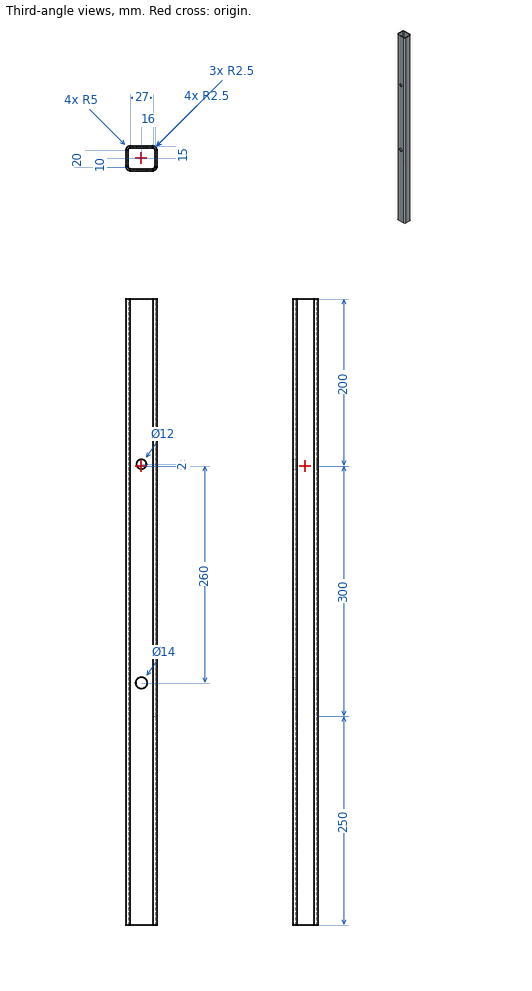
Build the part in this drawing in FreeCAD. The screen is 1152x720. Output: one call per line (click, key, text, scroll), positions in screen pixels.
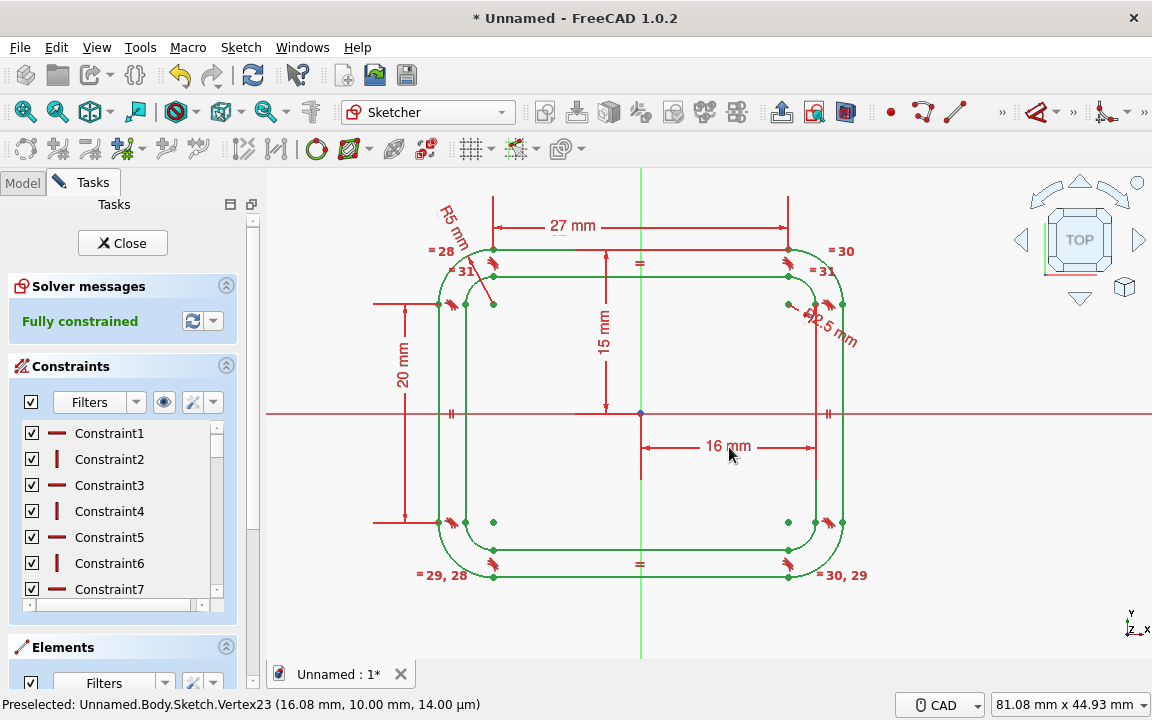
click(123, 243)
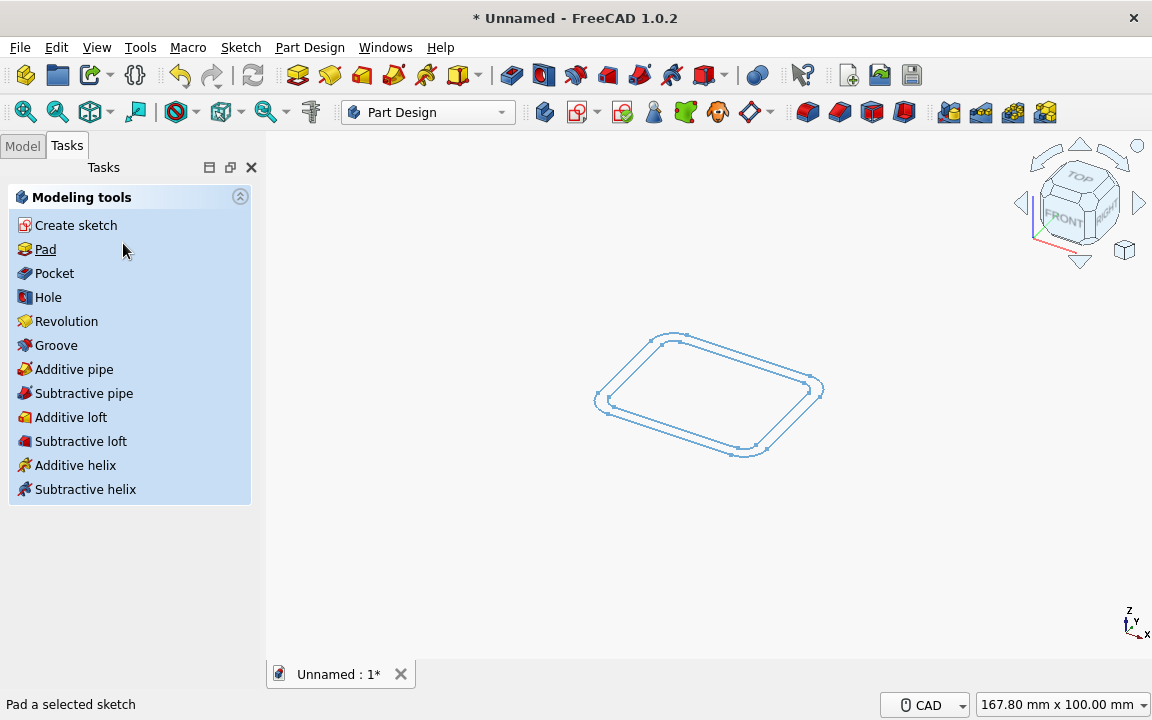
click(298, 76)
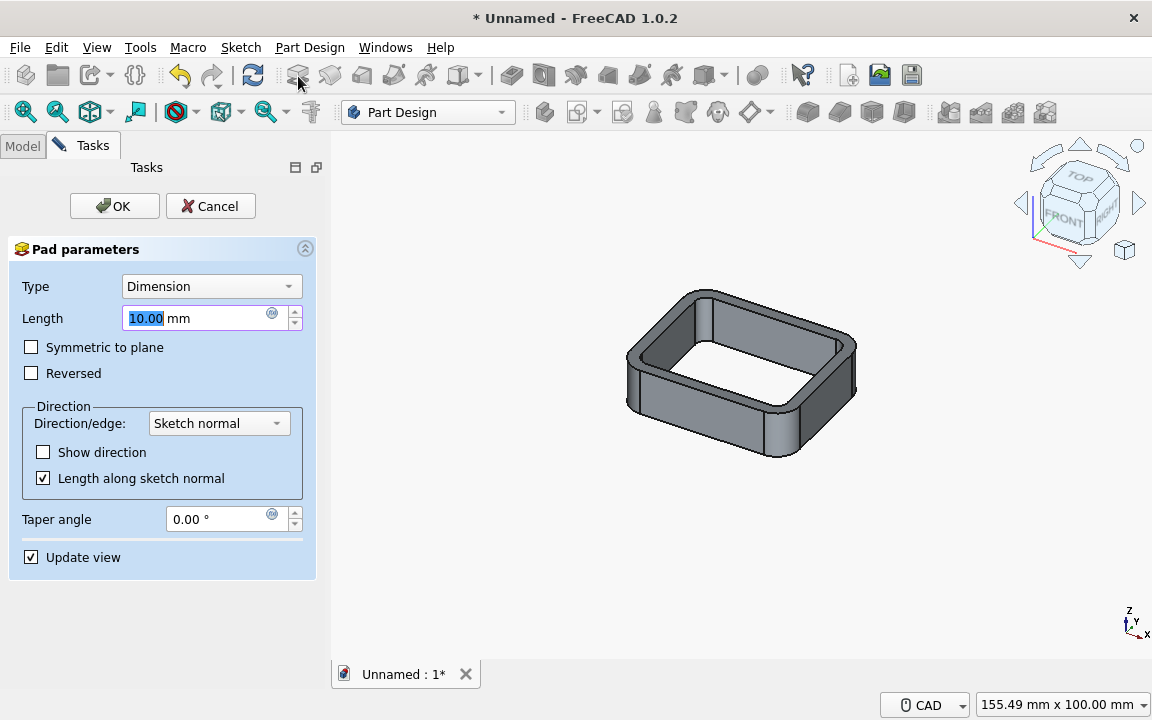
click(212, 286)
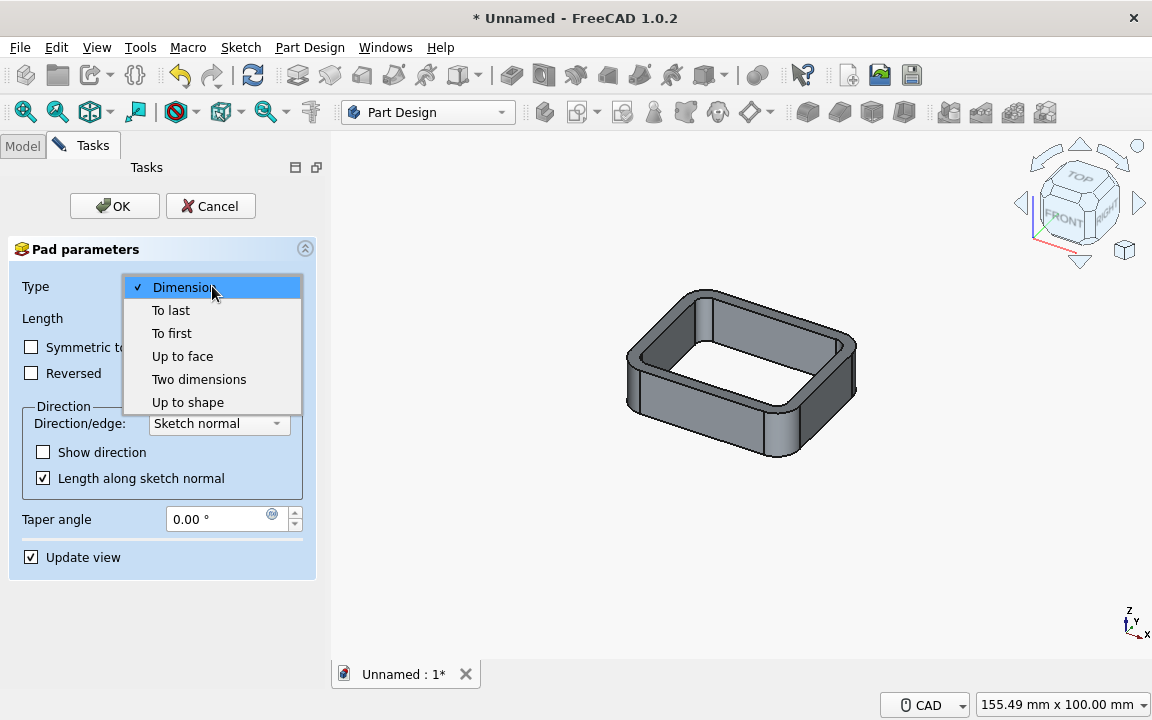
click(212, 380)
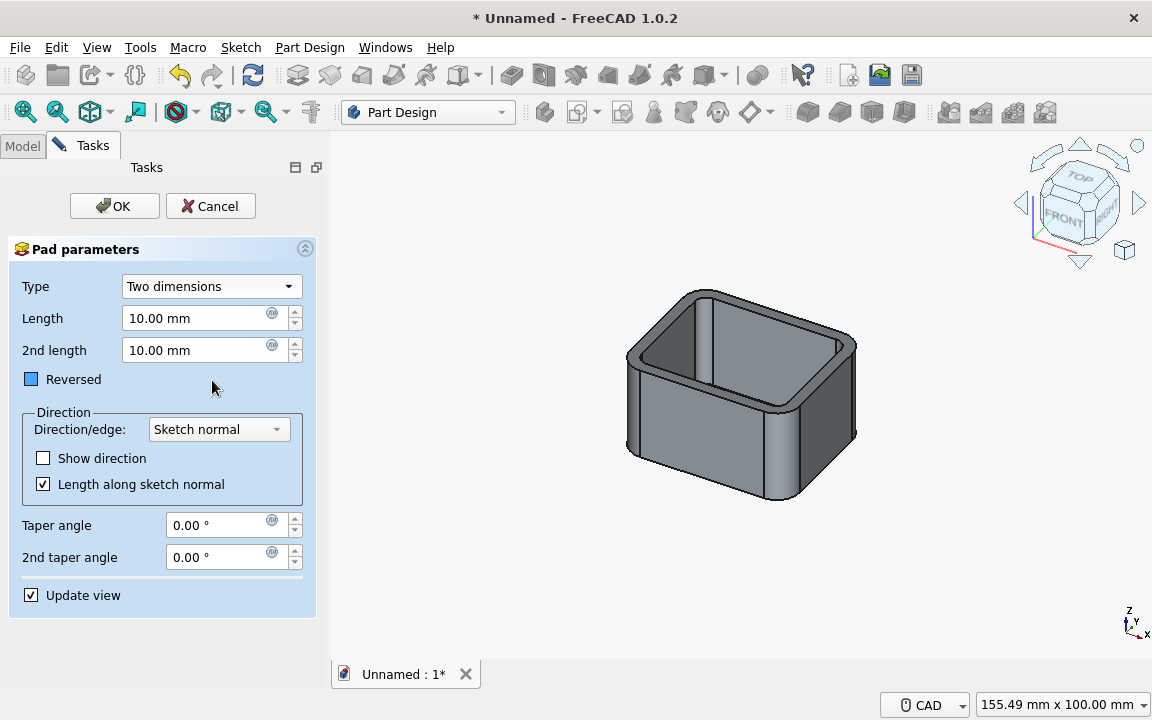
triple_click(204, 318)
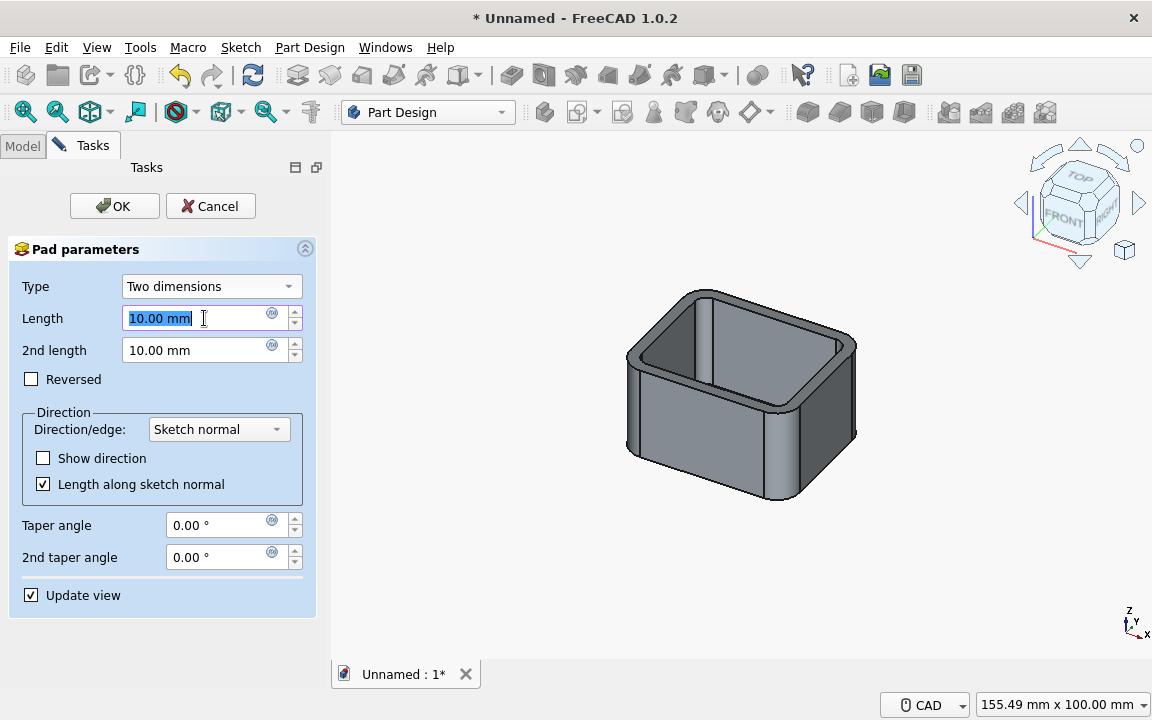
text(200)
key(Tab)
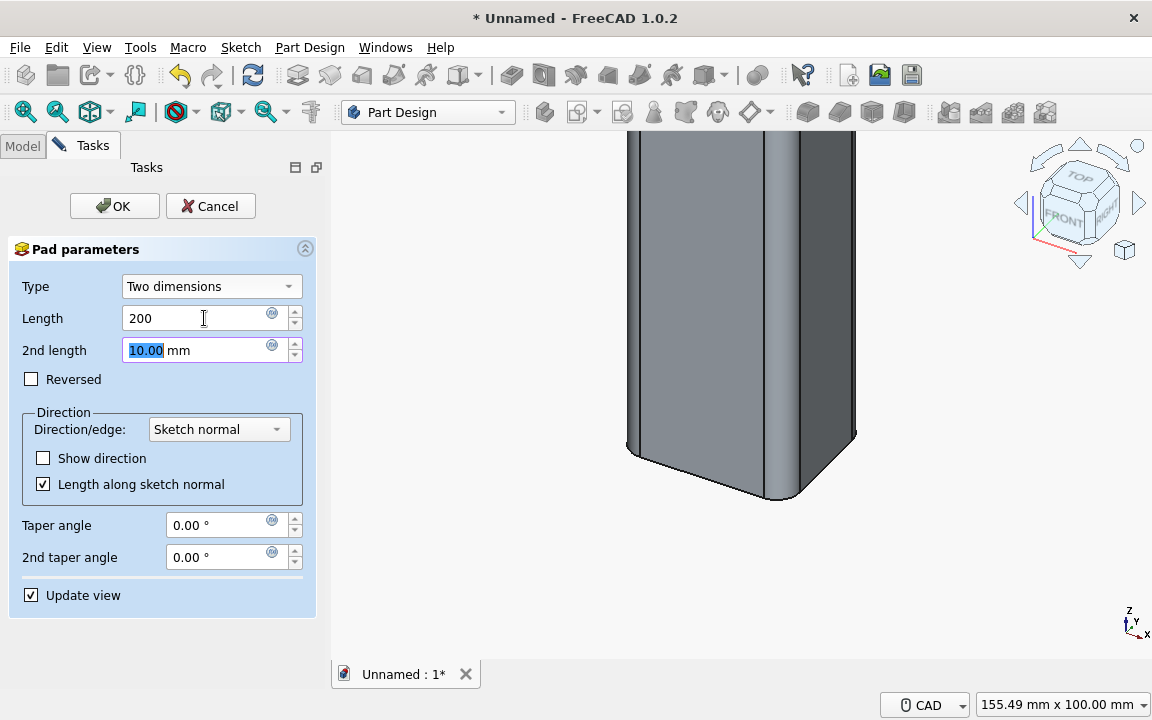
text(300)
key(Tab)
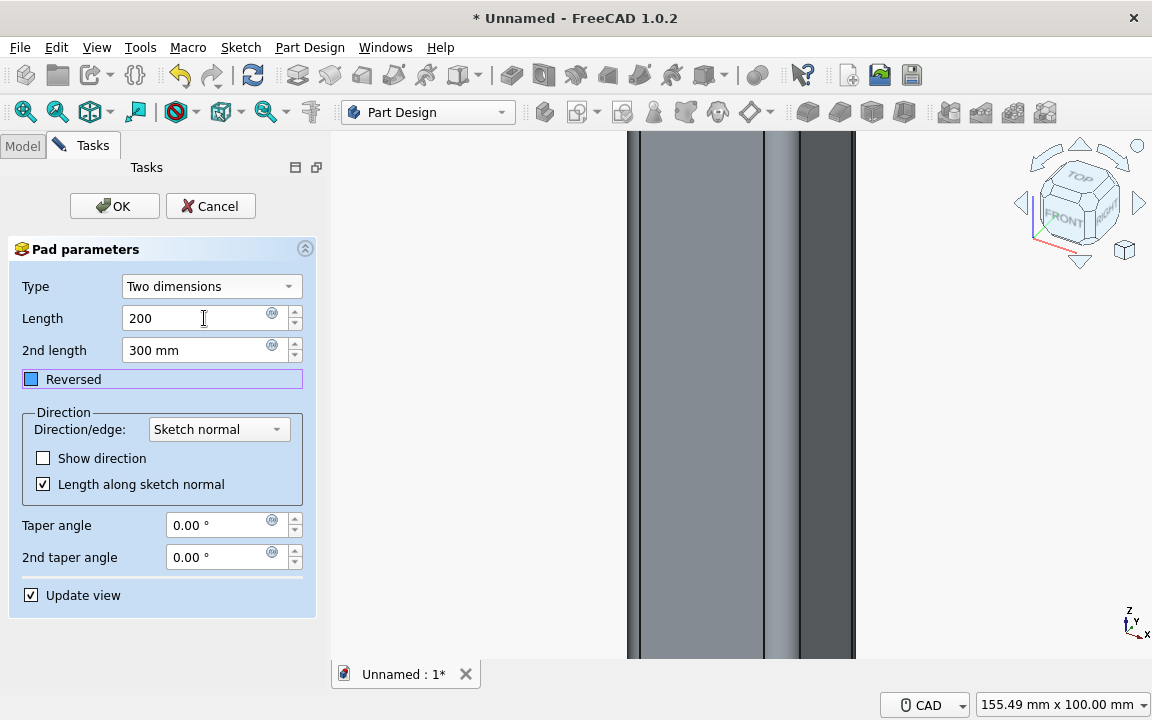
click(115, 206)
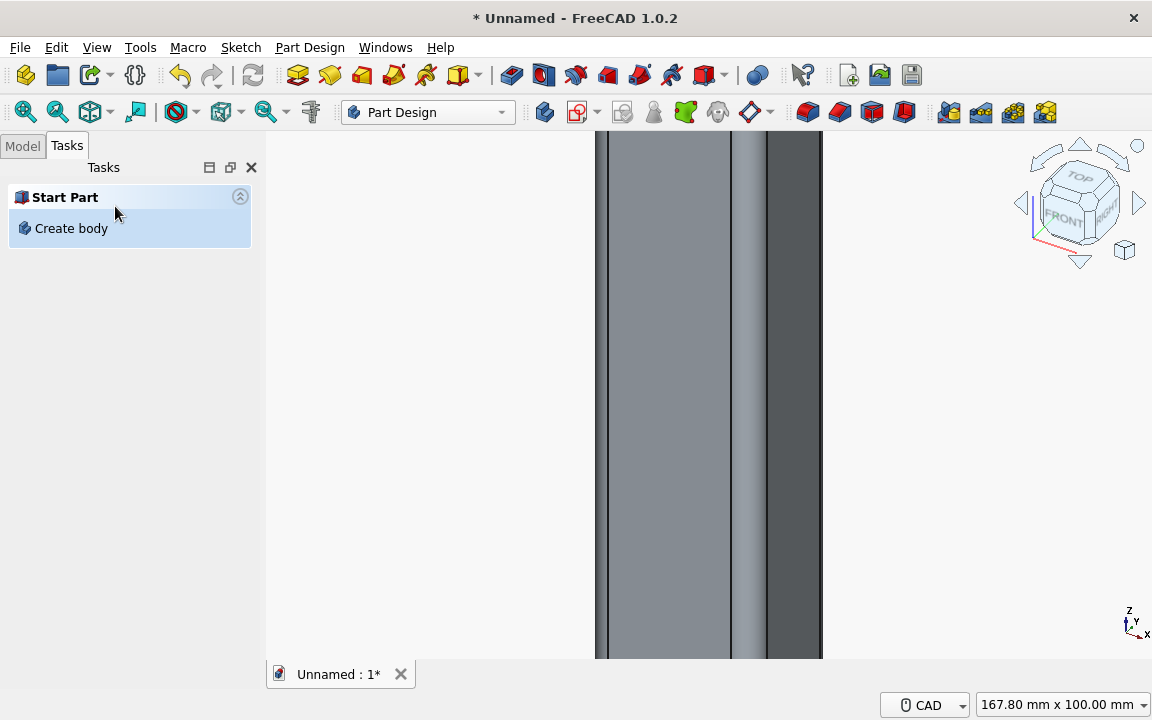
key(v)
key(f)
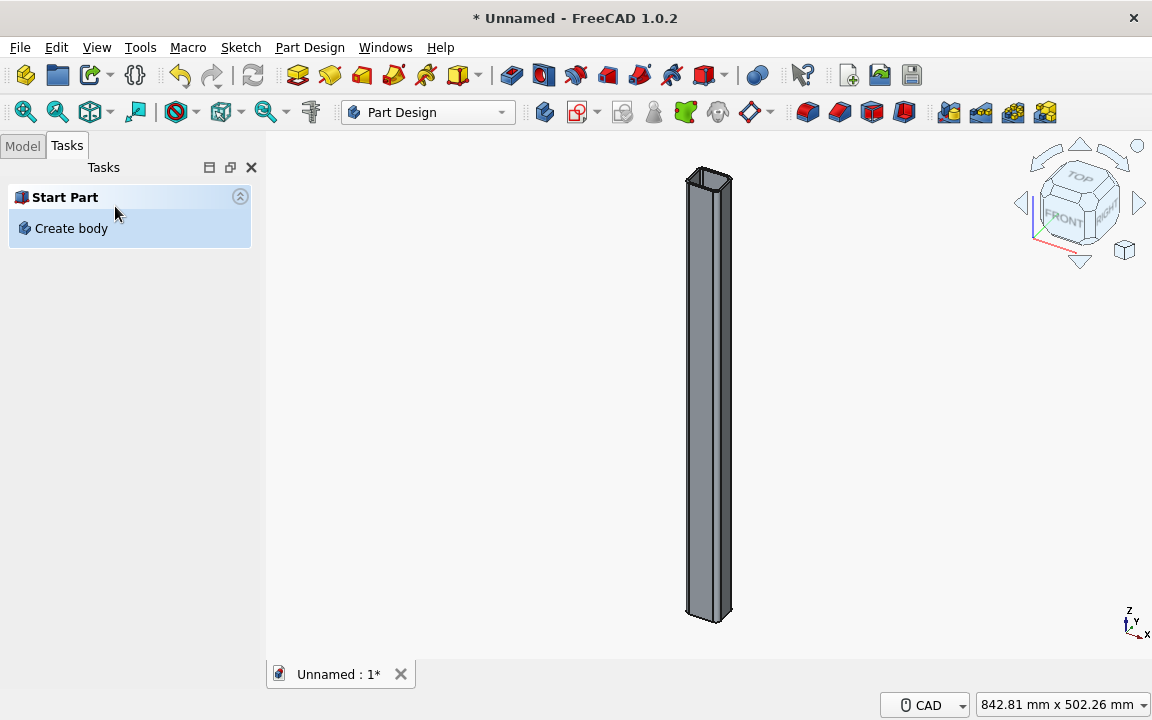
key(4)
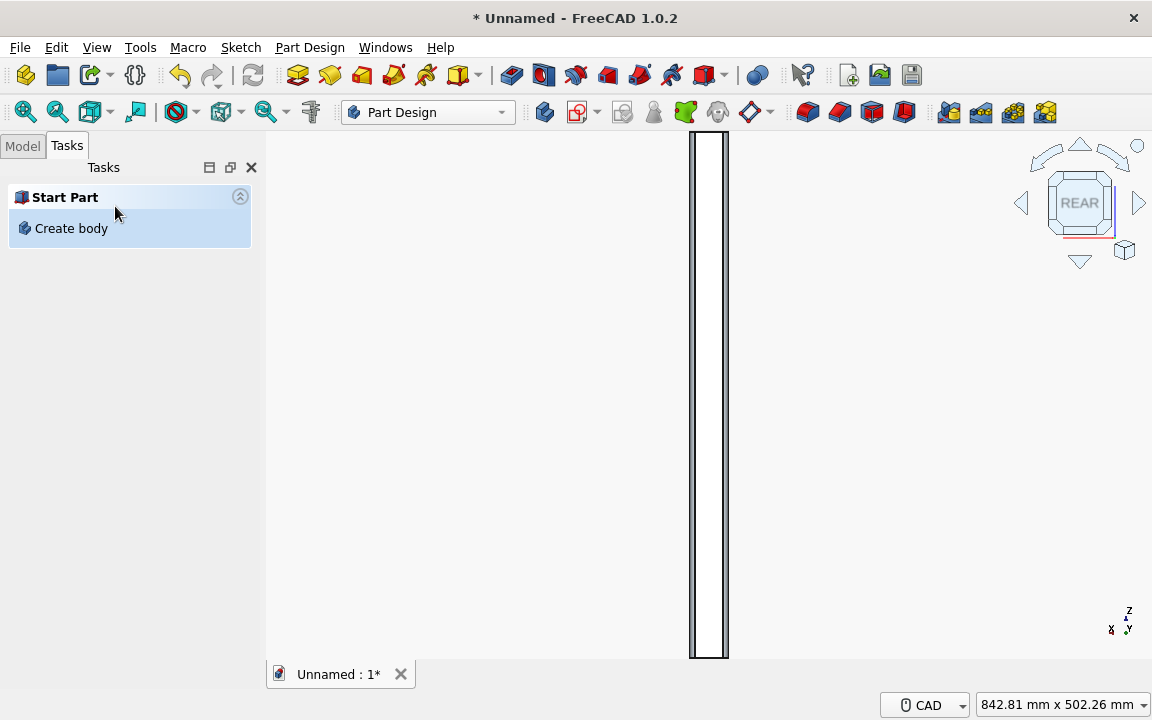
click(709, 169)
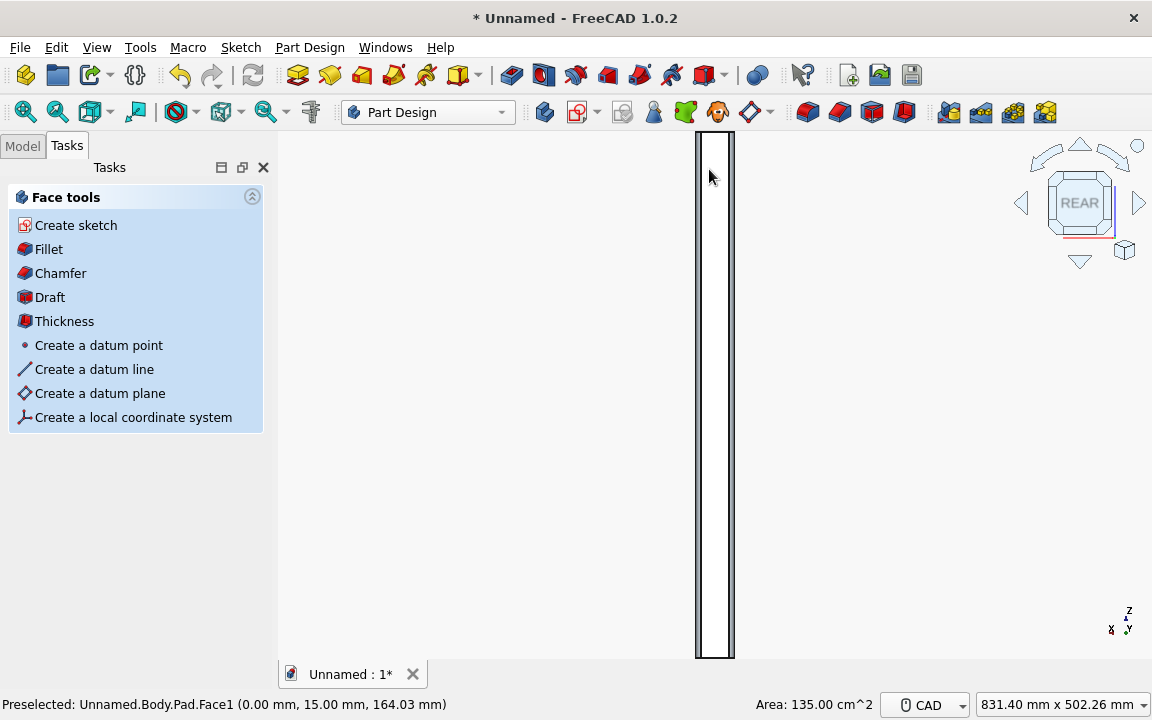
click(578, 112)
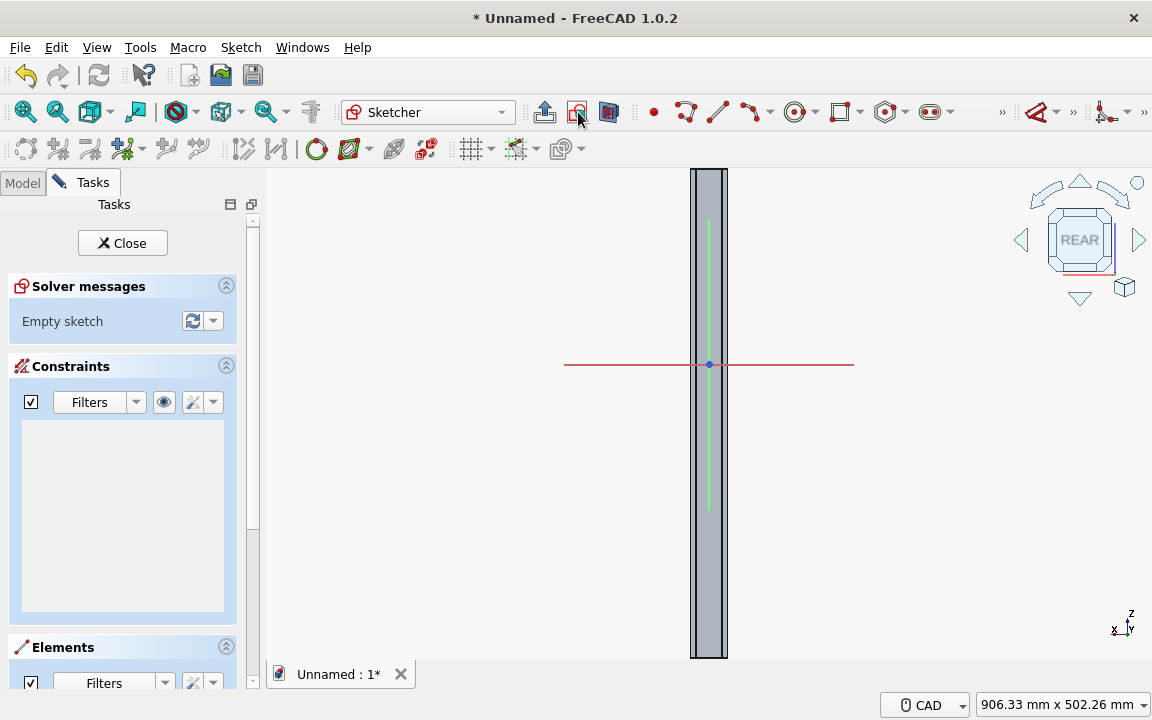
scroll(713, 360, up, 15)